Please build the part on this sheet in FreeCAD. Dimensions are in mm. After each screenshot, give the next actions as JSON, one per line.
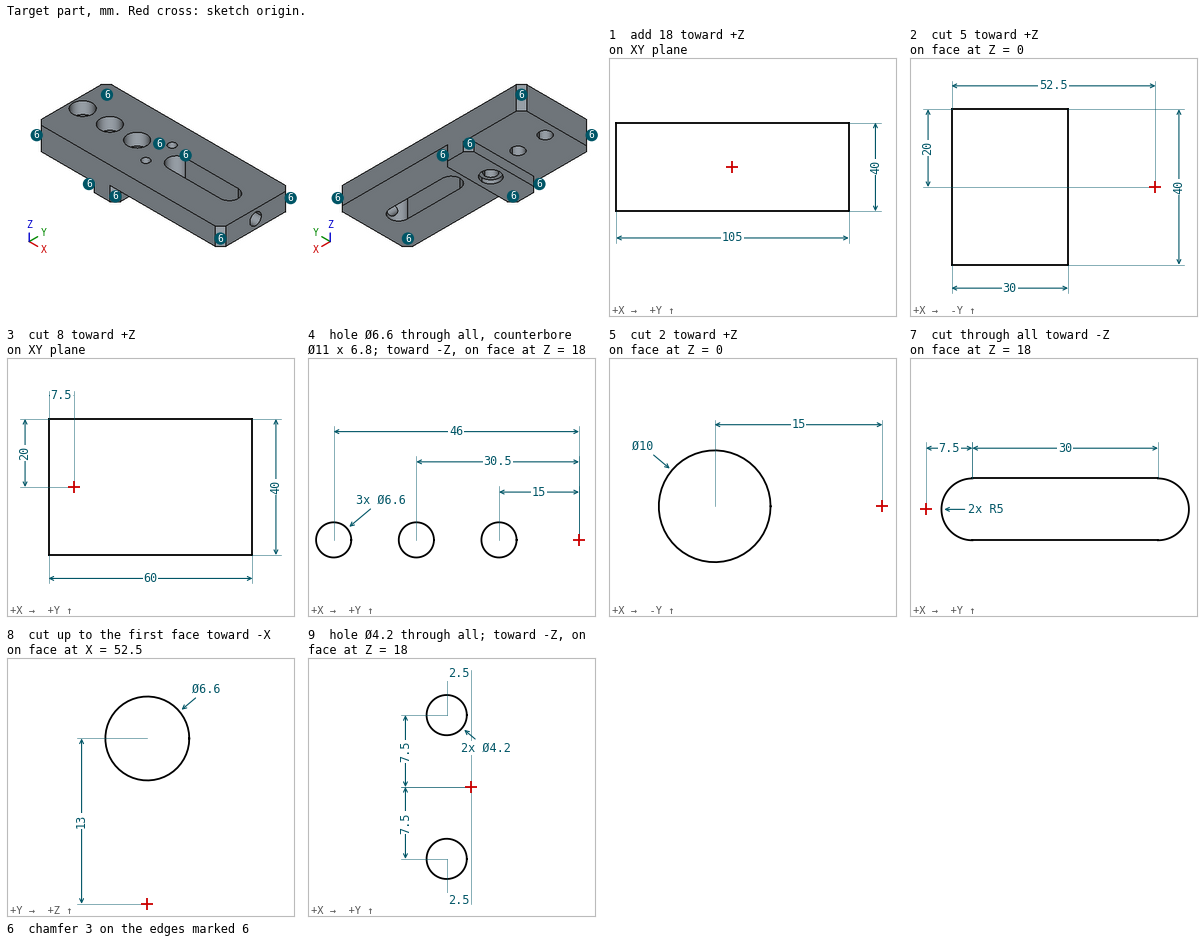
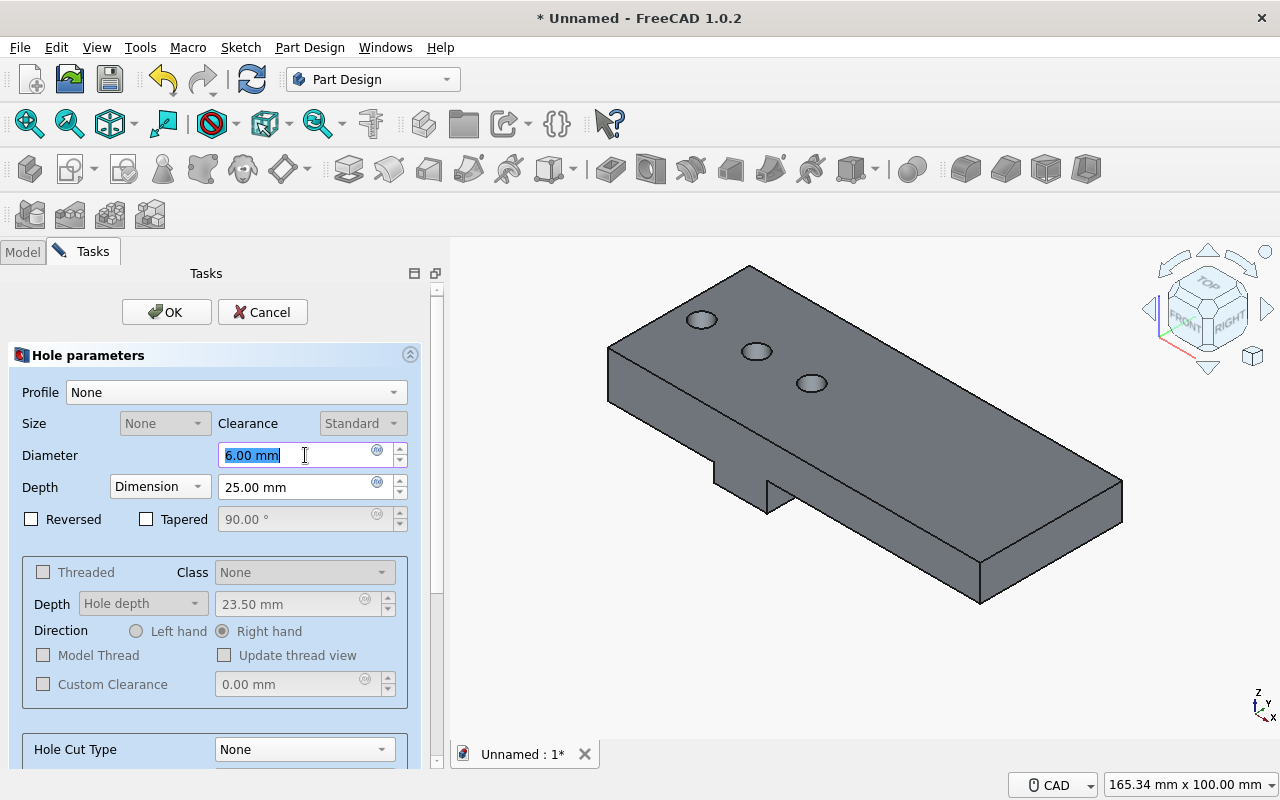
{"action": "type", "text": "6.6"}
{"action": "key", "text": "Tab"}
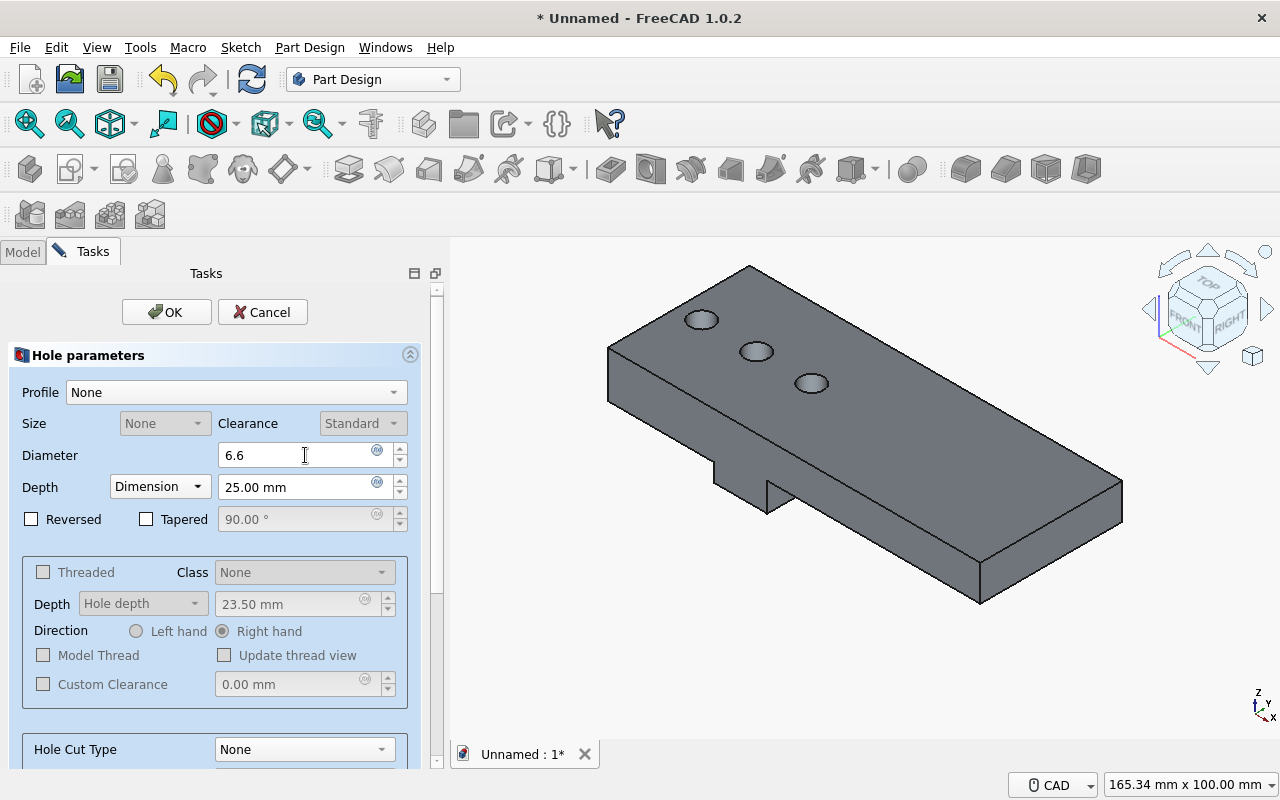
{"action": "left_click", "coordinate": [161, 486]}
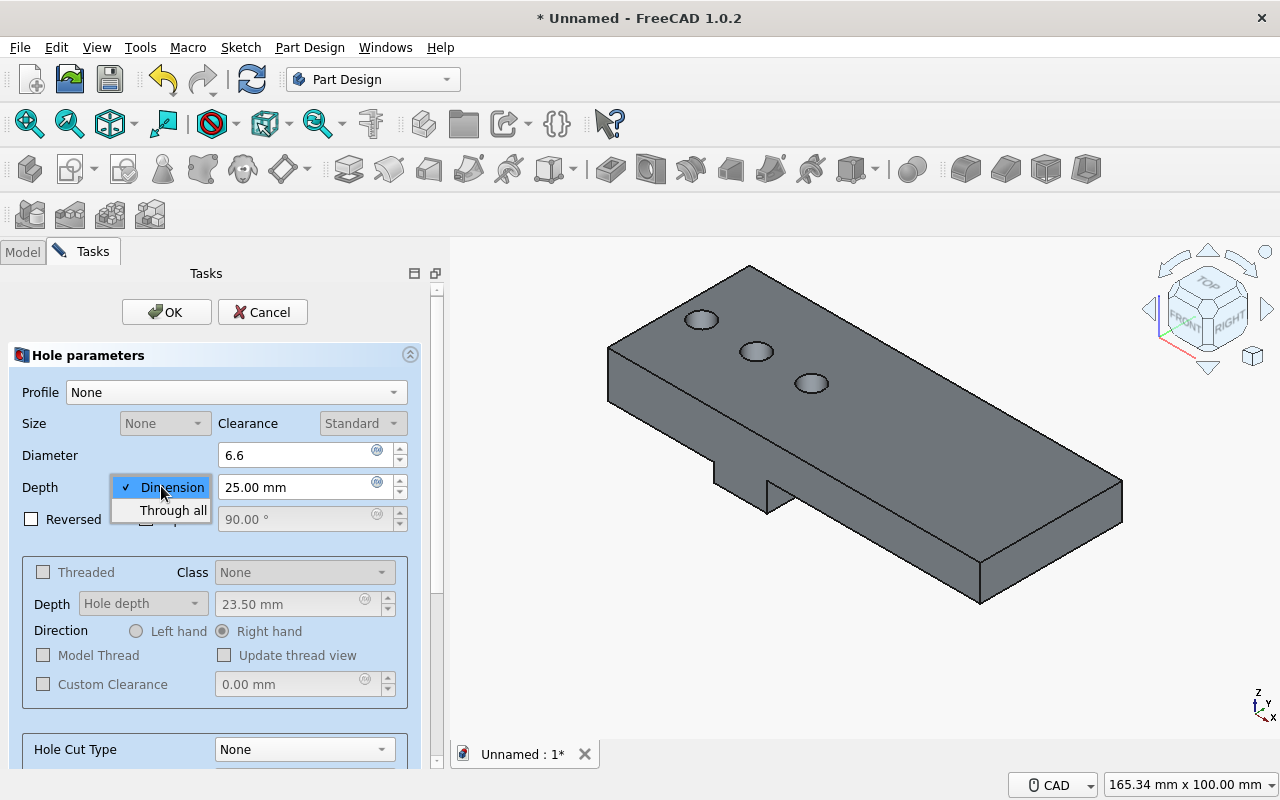
{"action": "left_click", "coordinate": [160, 510]}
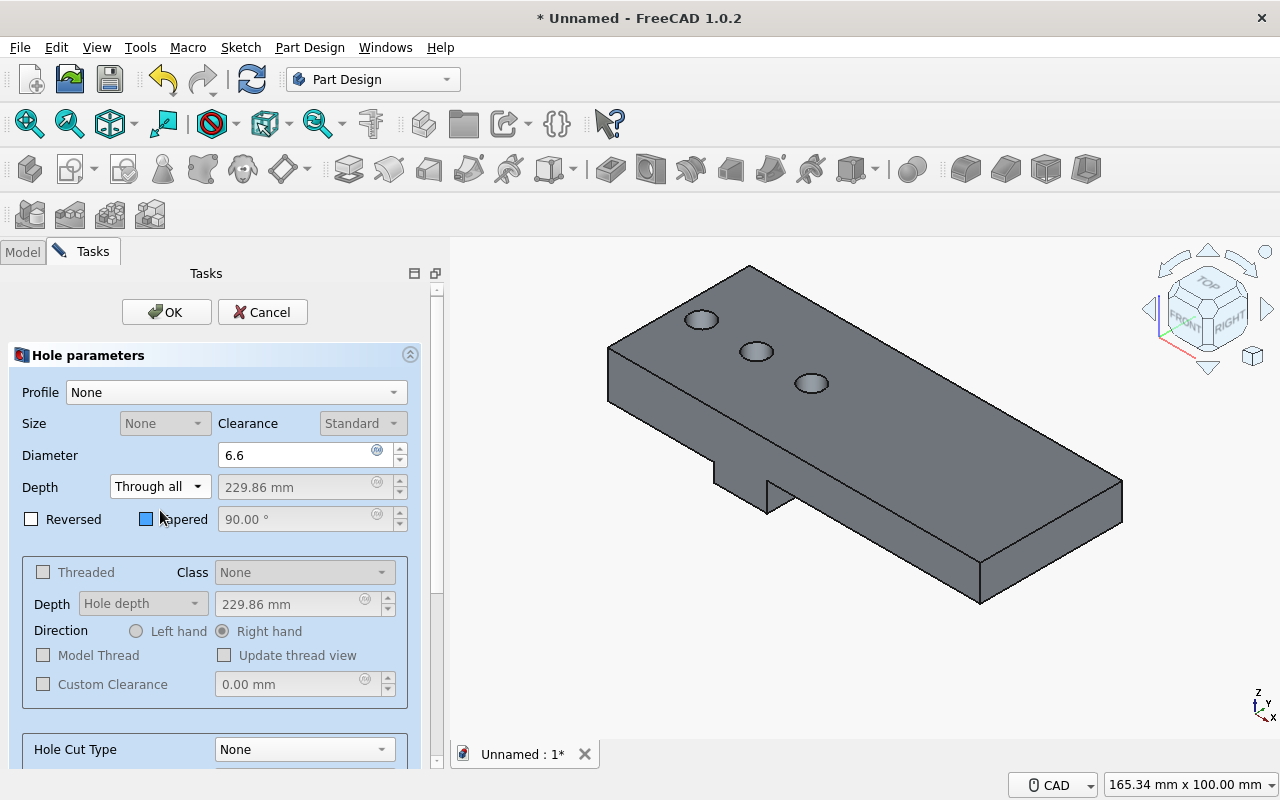
{"action": "left_click", "coordinate": [306, 750]}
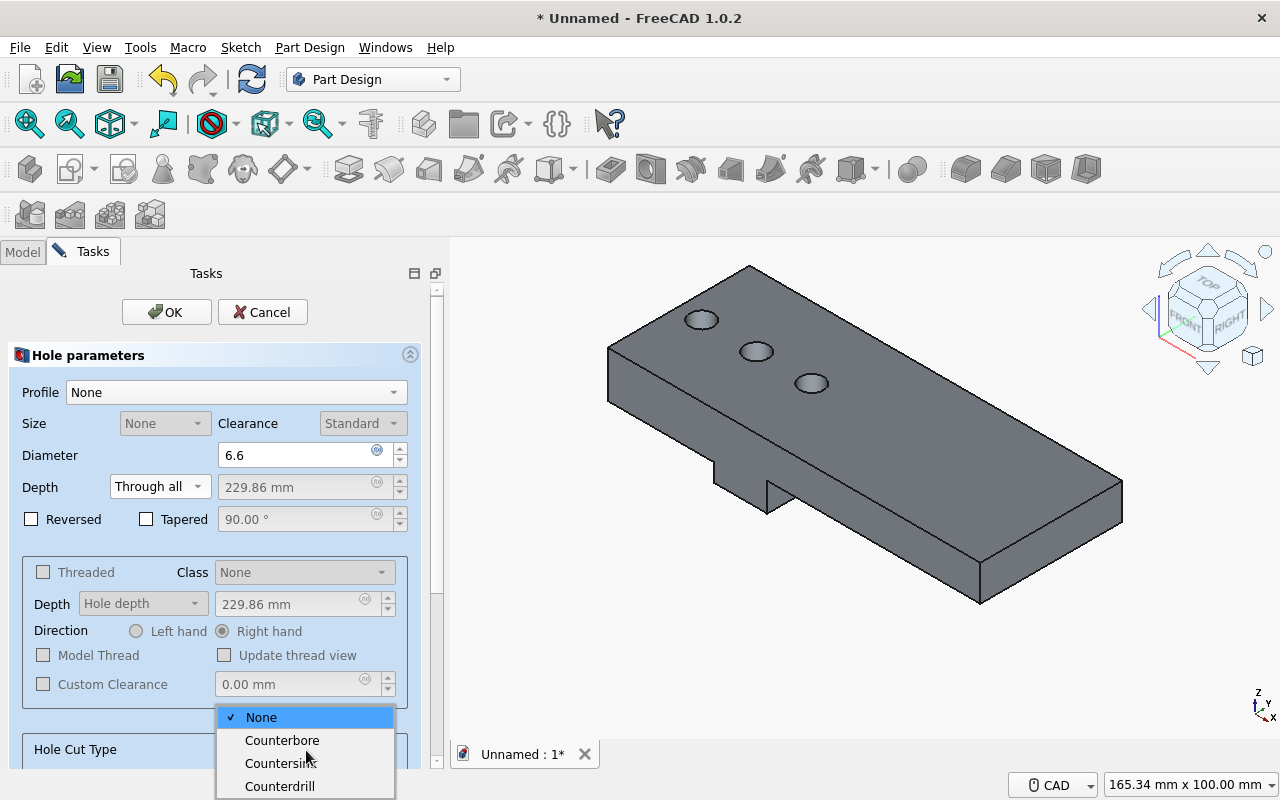
{"action": "left_click", "coordinate": [304, 740]}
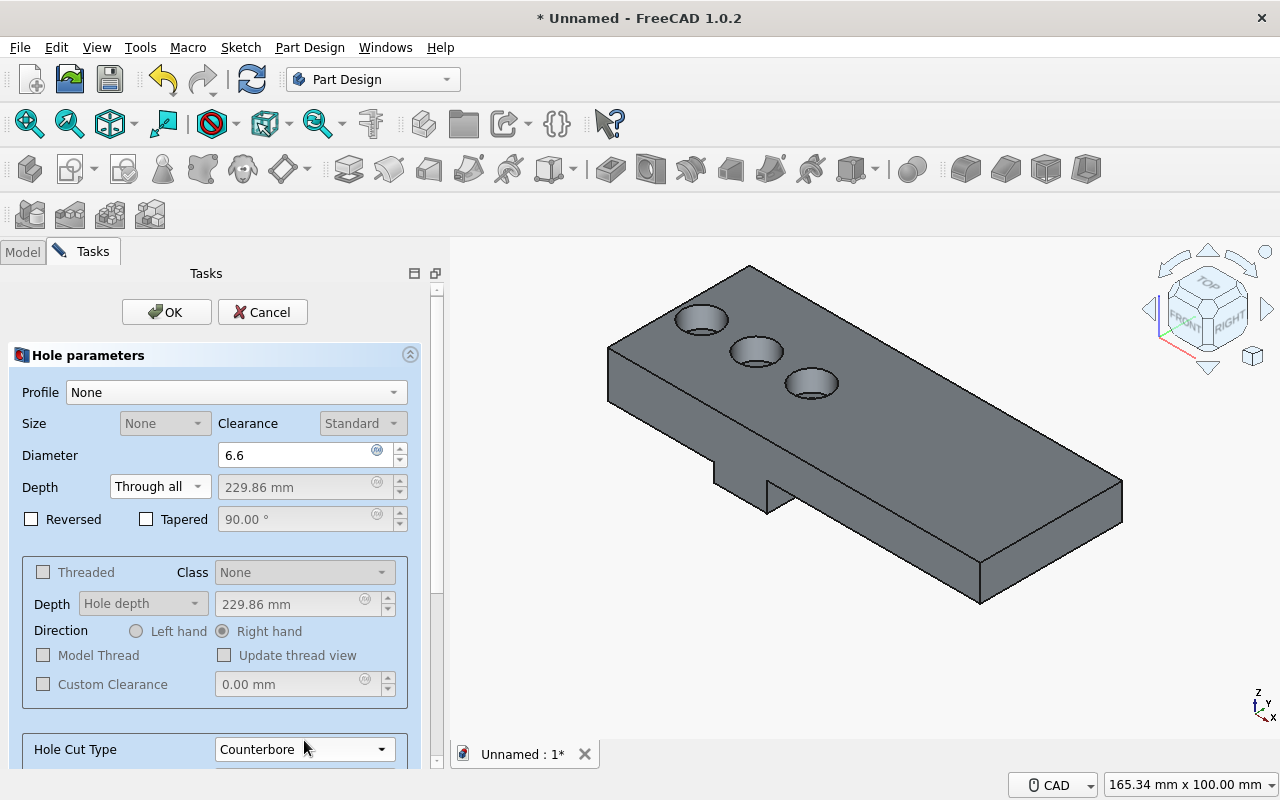
{"action": "scroll", "coordinate": [437, 526], "scroll_direction": "down", "scroll_amount": 2}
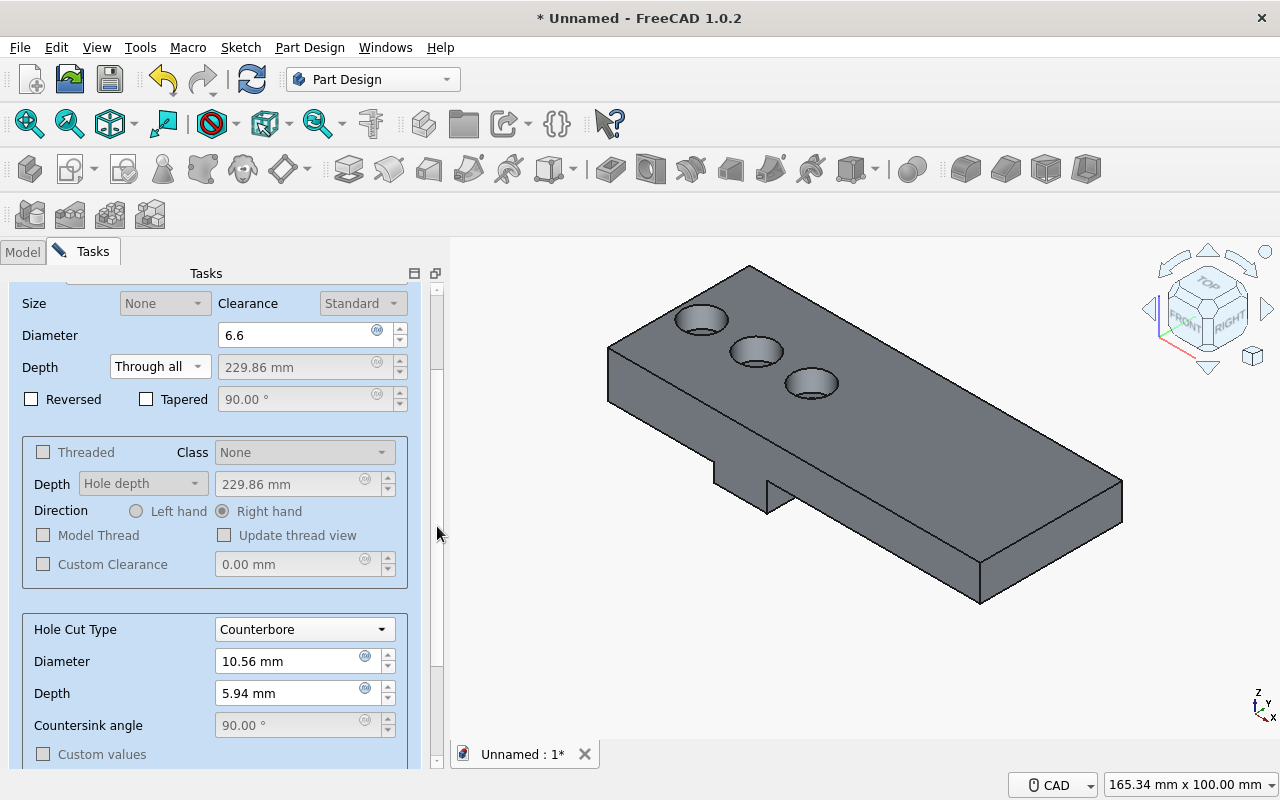
{"action": "triple_click", "coordinate": [298, 661]}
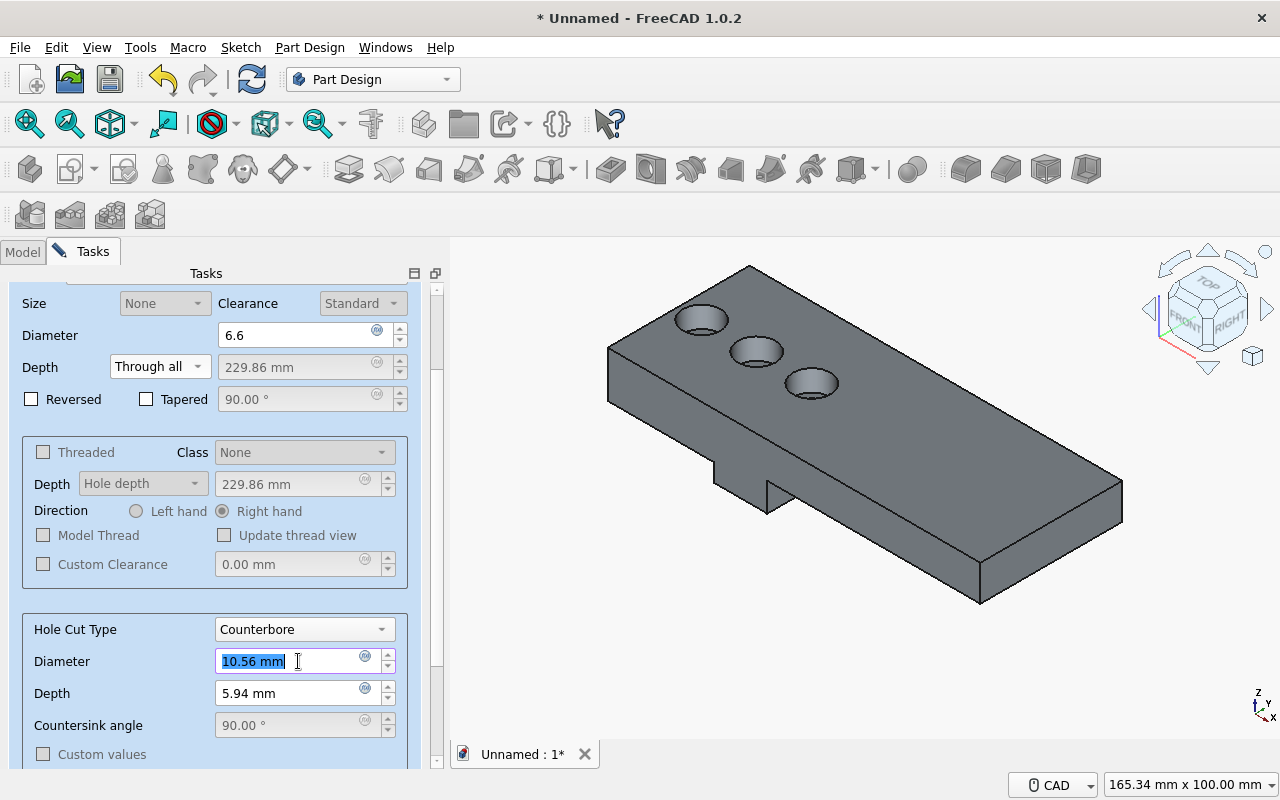
{"action": "type", "text": "11"}
{"action": "key", "text": "Tab"}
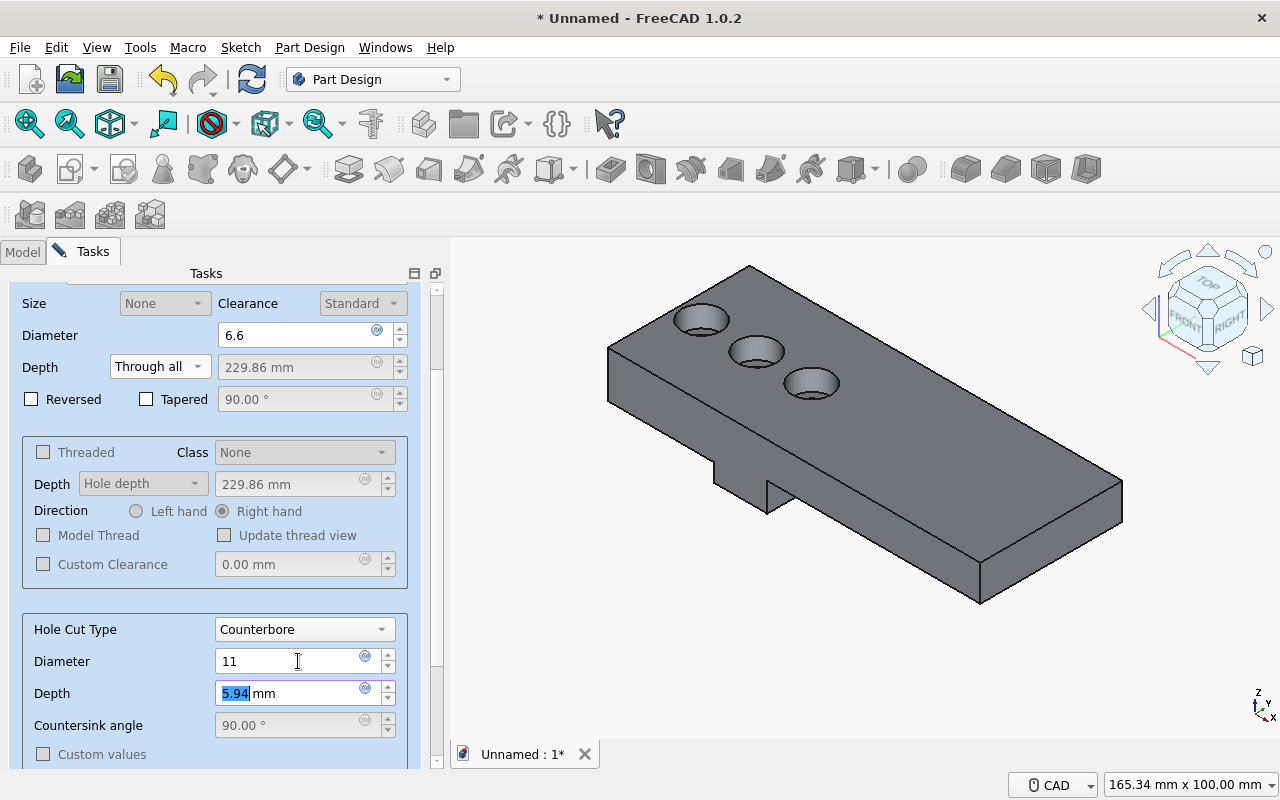
{"action": "type", "text": "6.8"}
{"action": "key", "text": "Tab"}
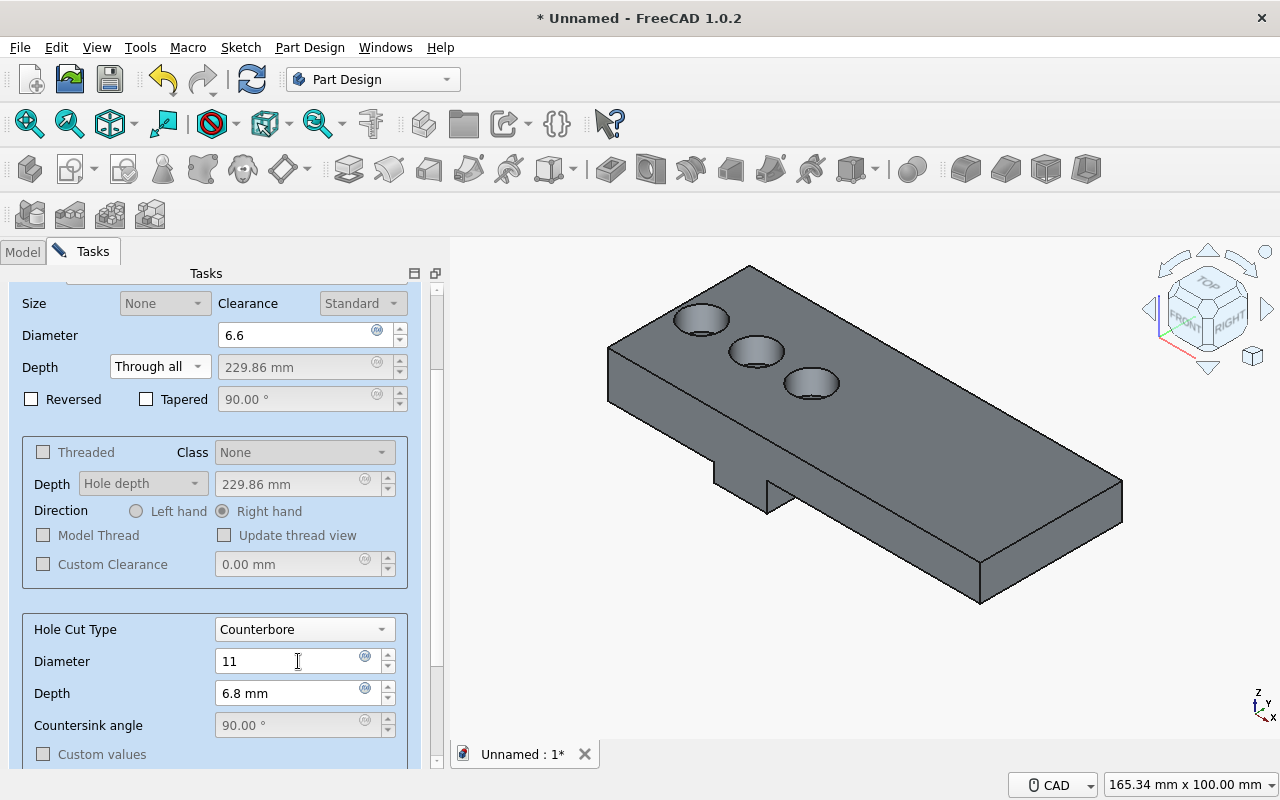
{"action": "scroll", "coordinate": [437, 526], "scroll_direction": "up", "scroll_amount": 3}